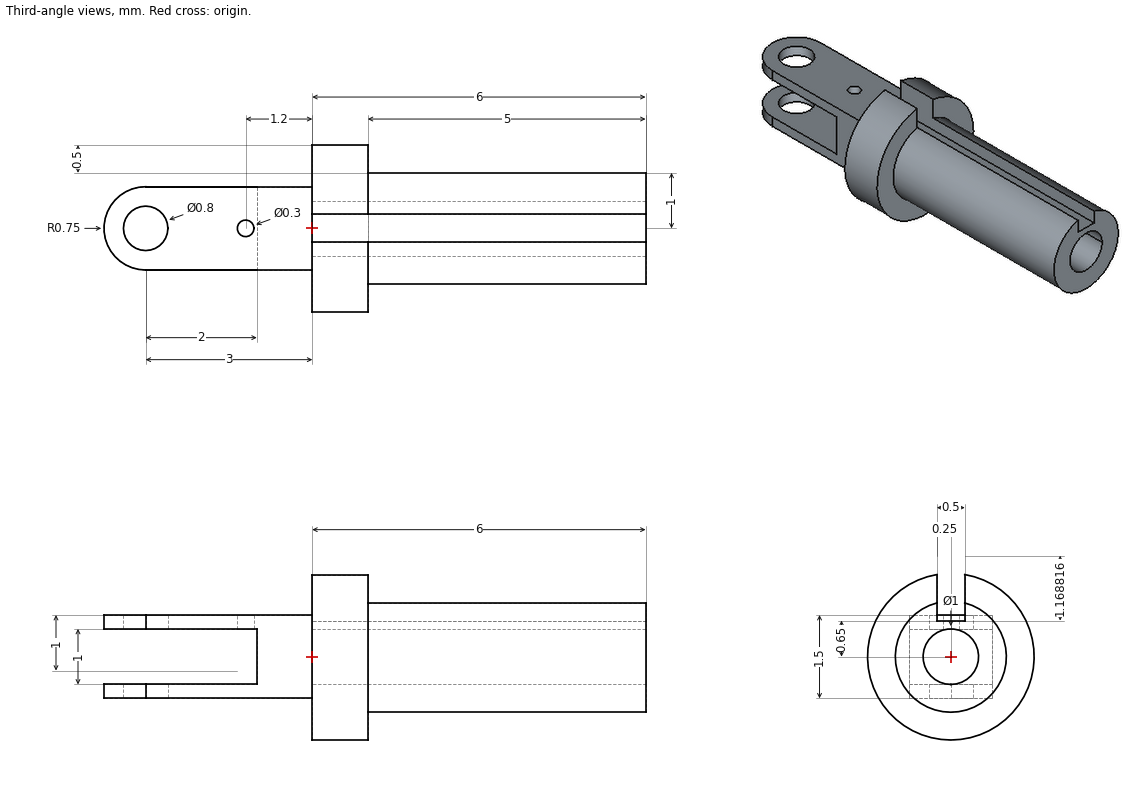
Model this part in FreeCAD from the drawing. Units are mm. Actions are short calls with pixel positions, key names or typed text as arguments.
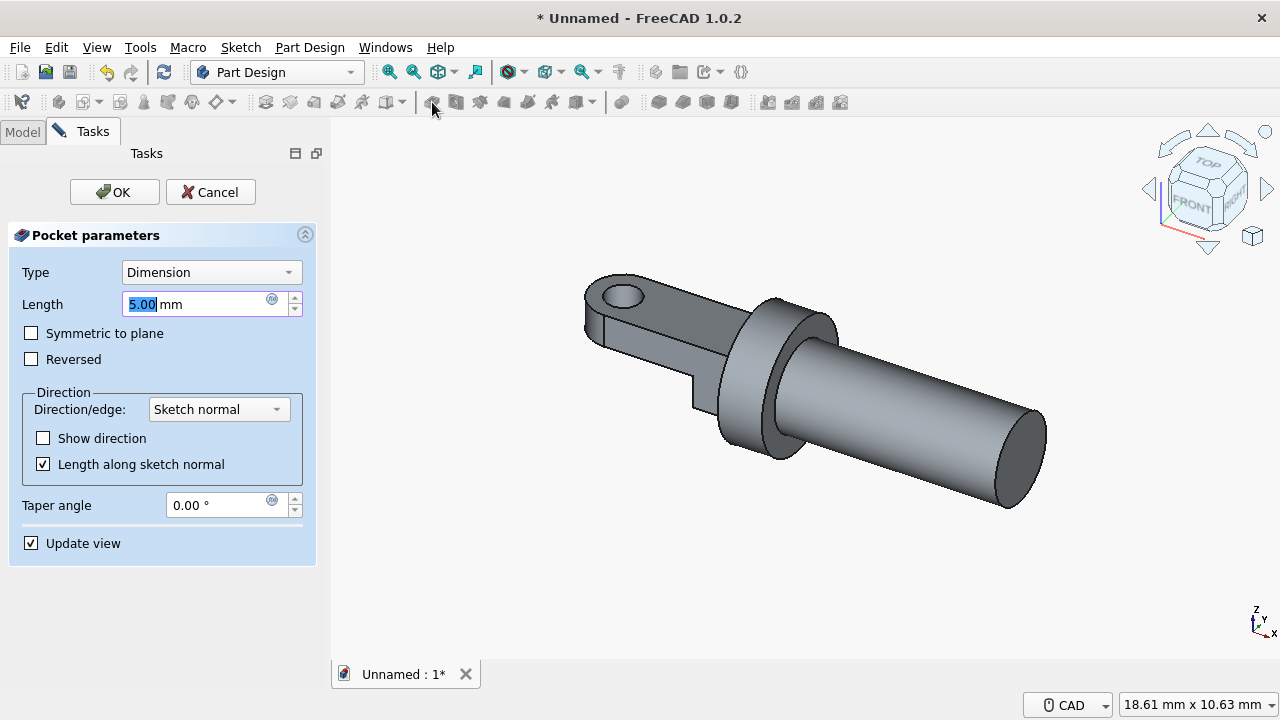
text(1)
key(Tab)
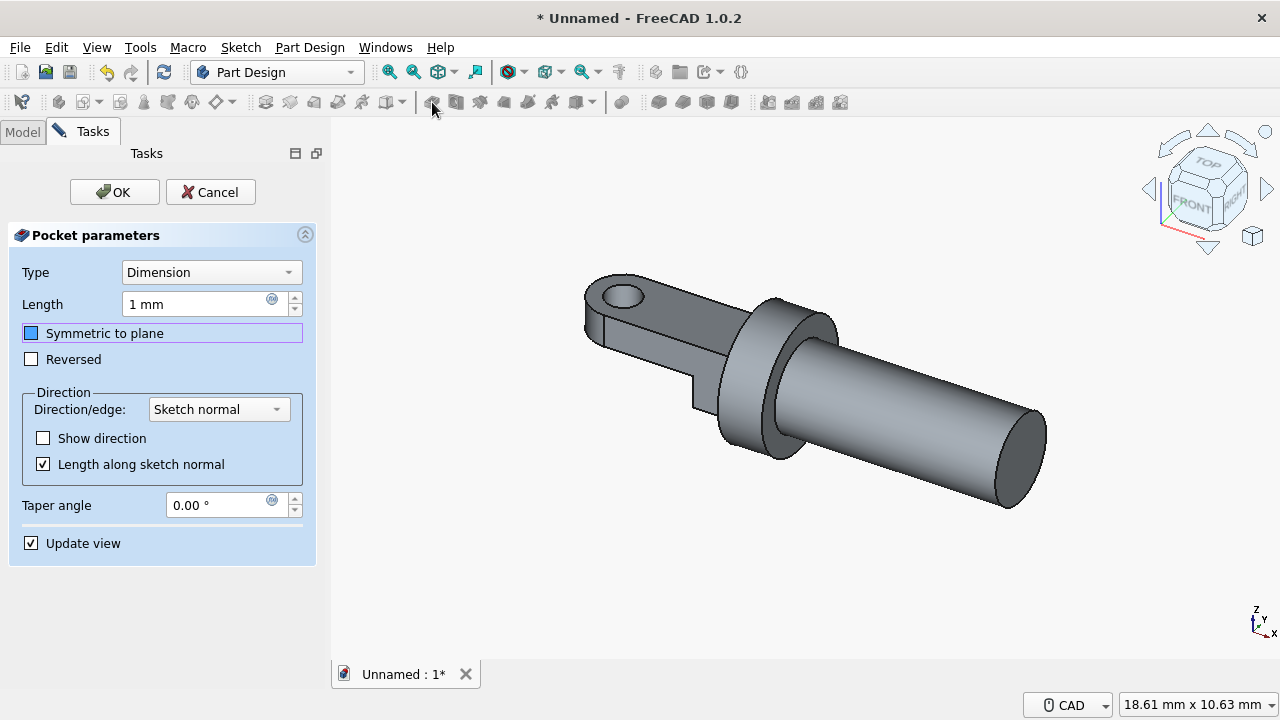
click(30, 333)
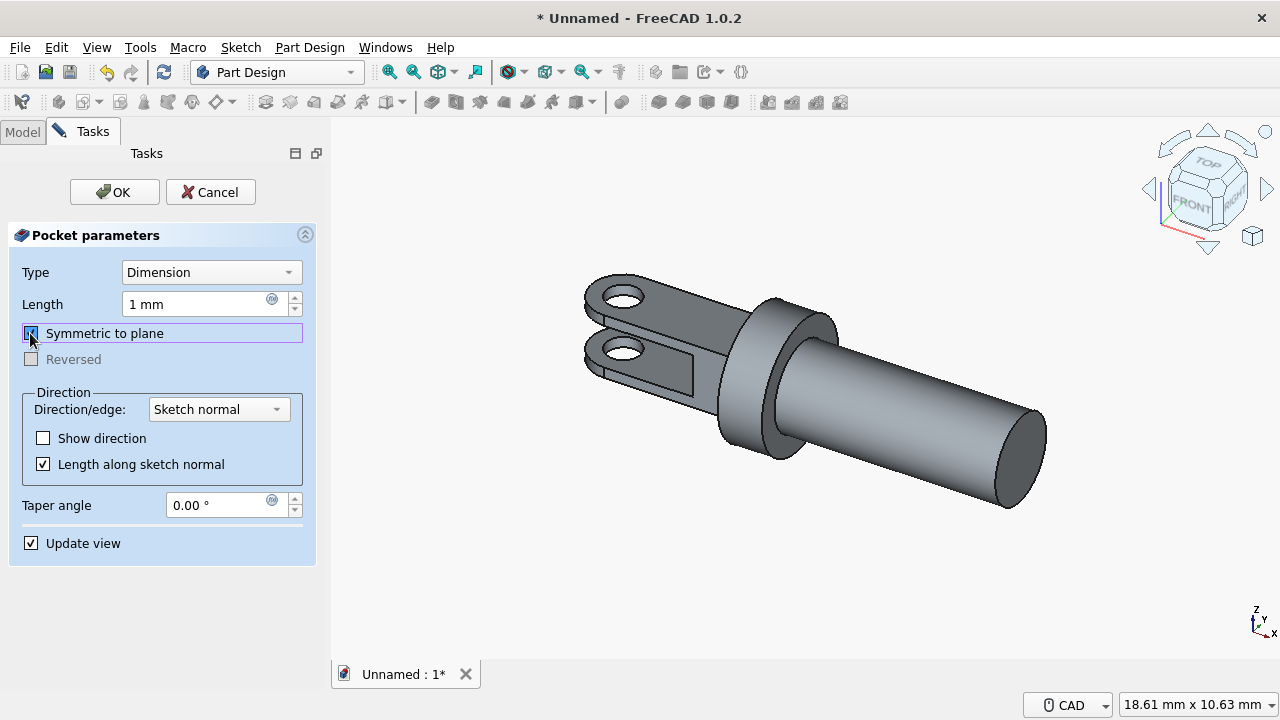
click(115, 192)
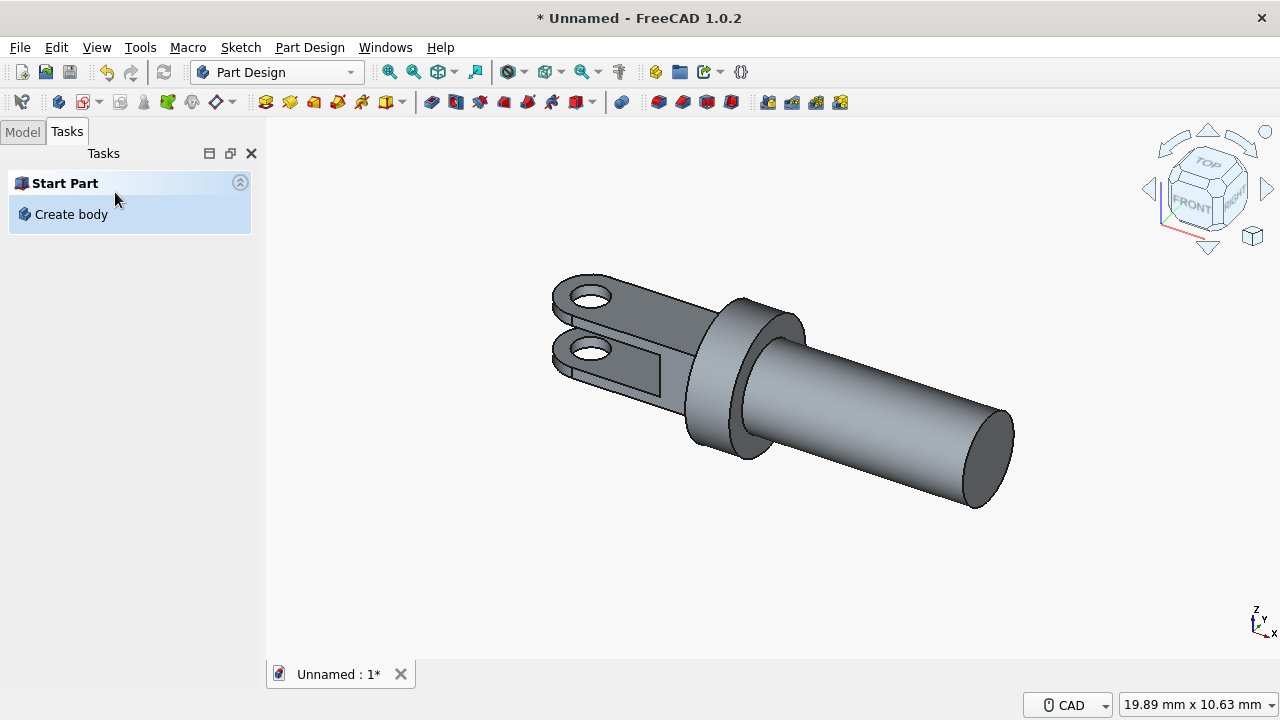
click(988, 458)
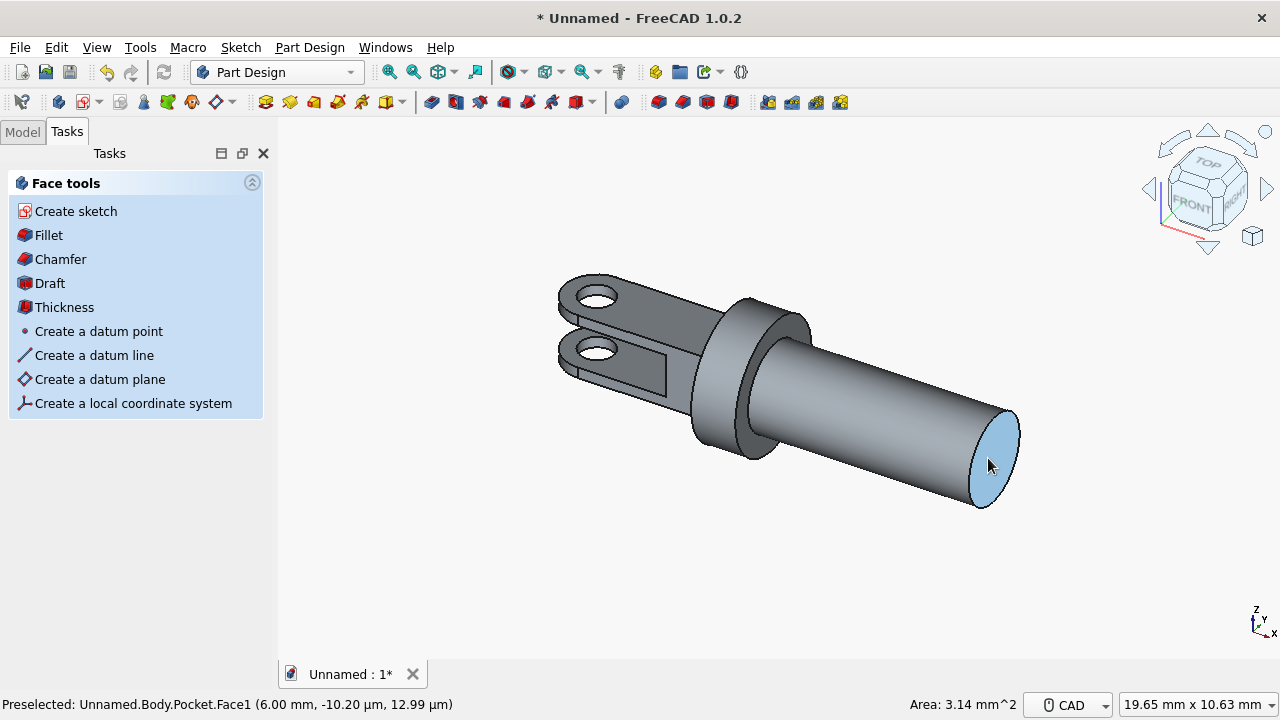
click(84, 102)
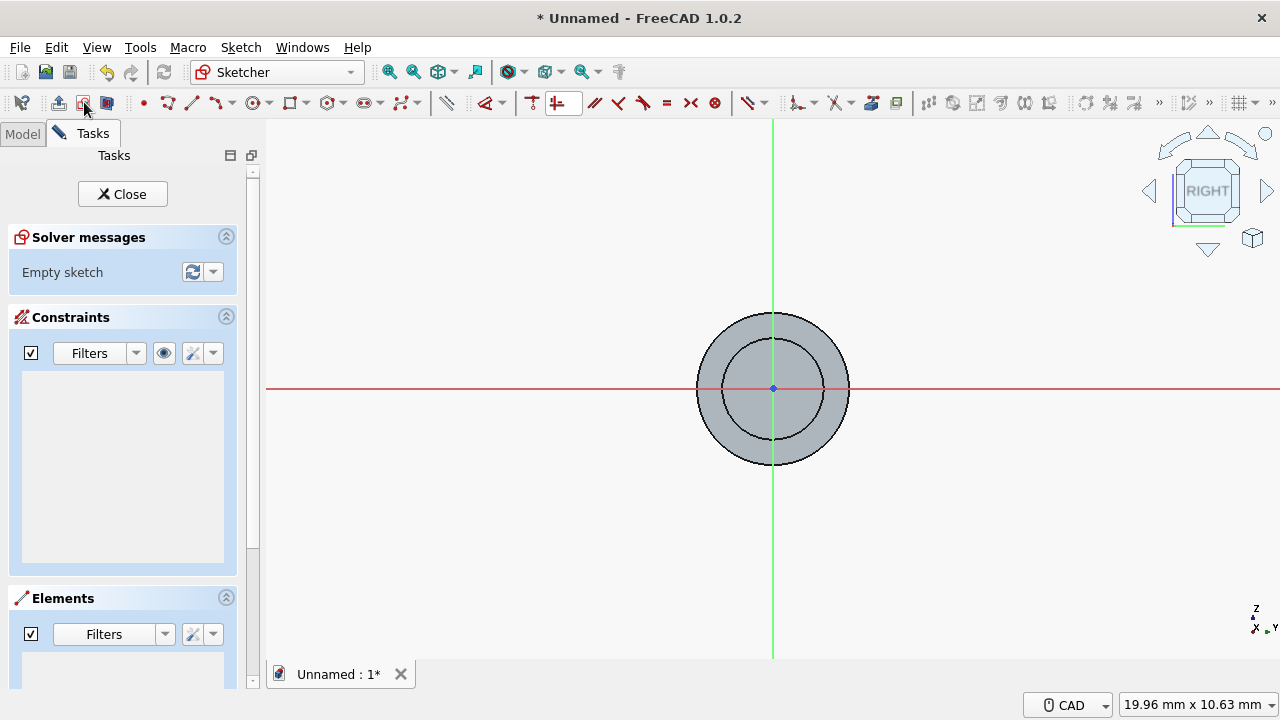
scroll(784, 389, up, 10)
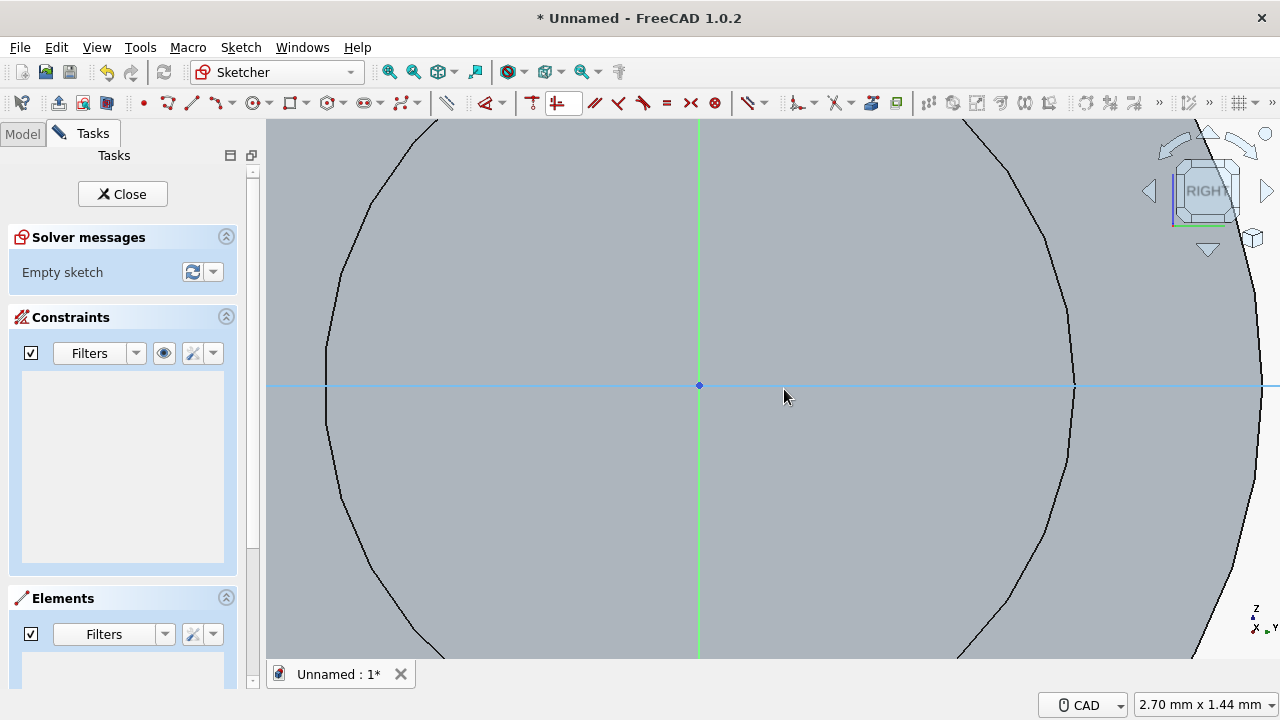
click(254, 104)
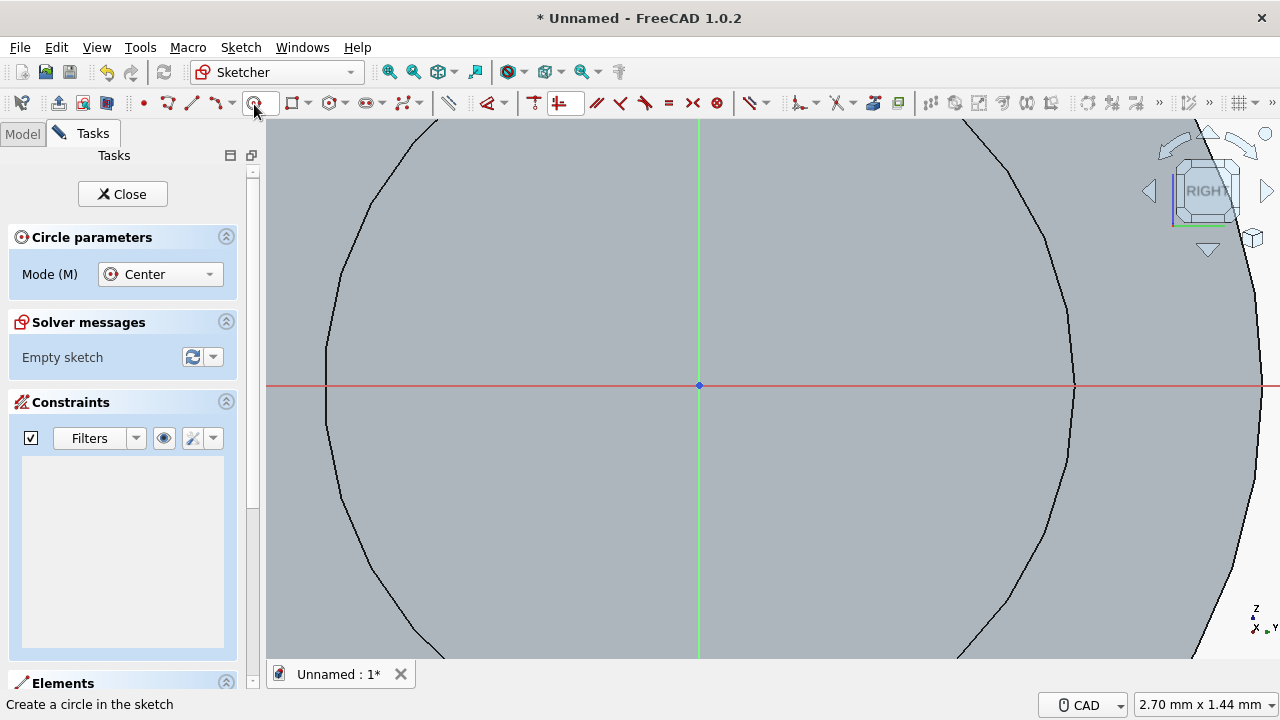
click(699, 386)
move(832, 253)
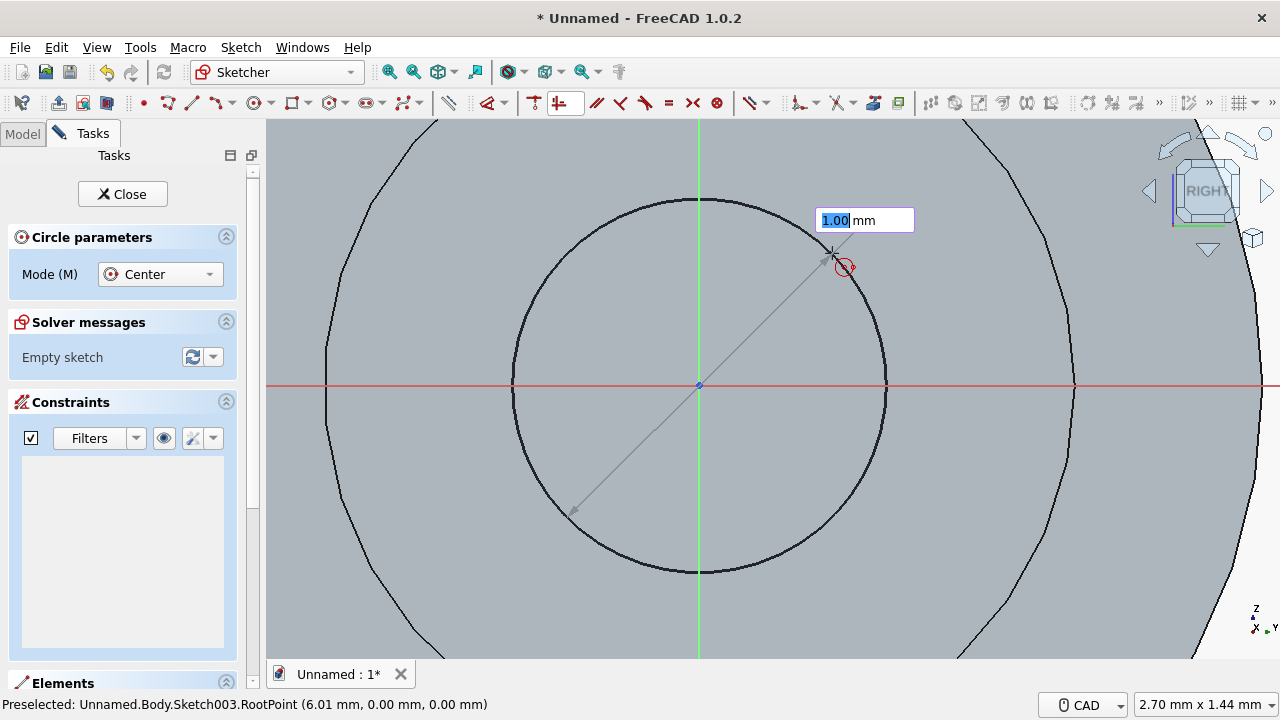
text(1)
key(Return)
key(Escape)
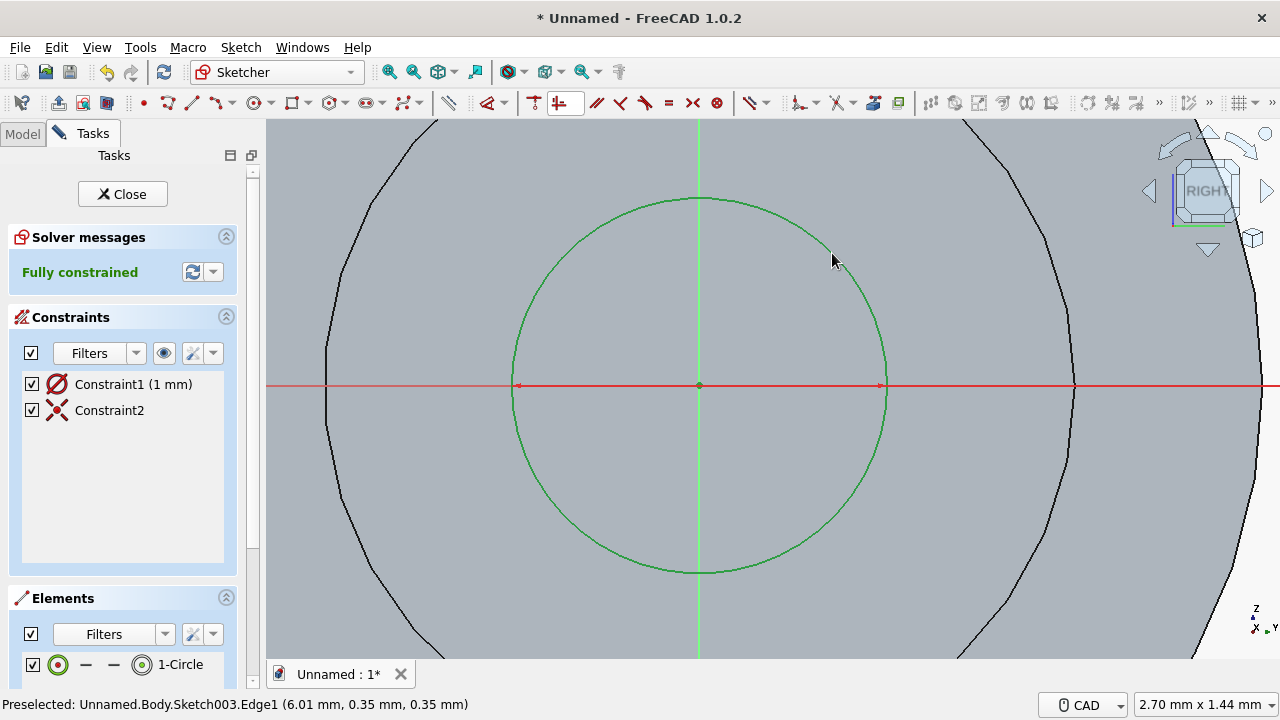
click(123, 194)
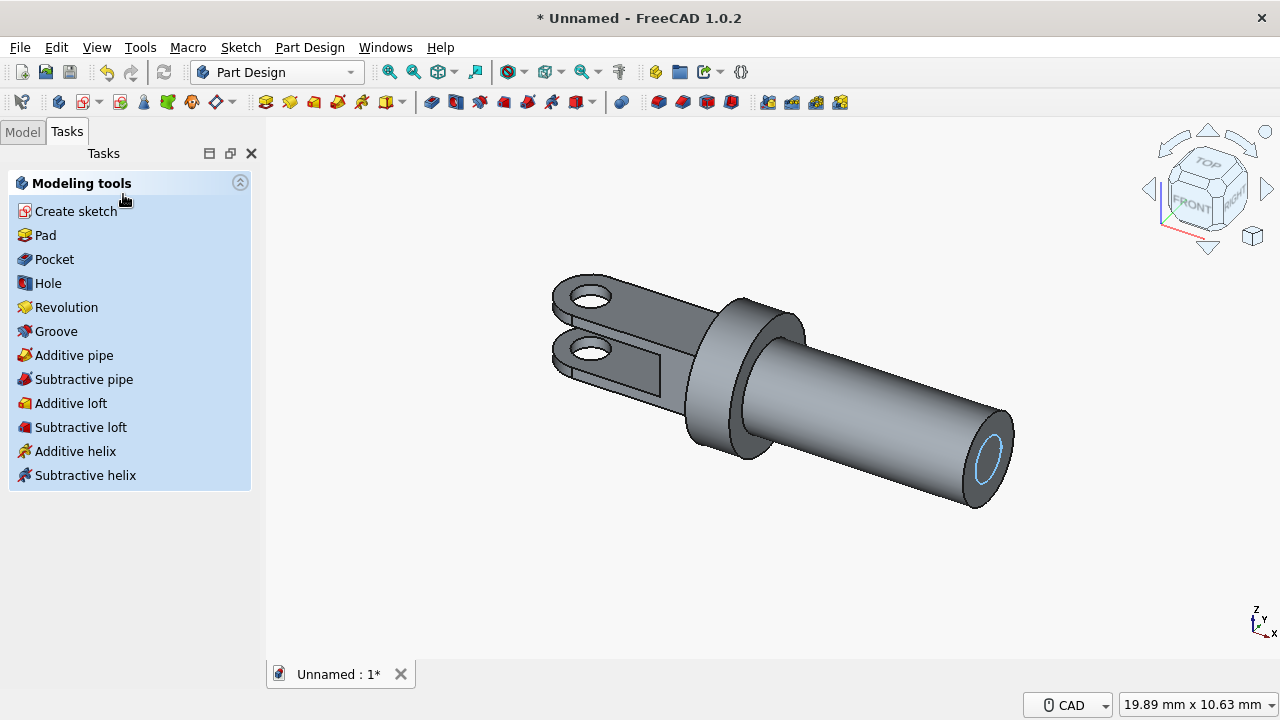
click(432, 102)